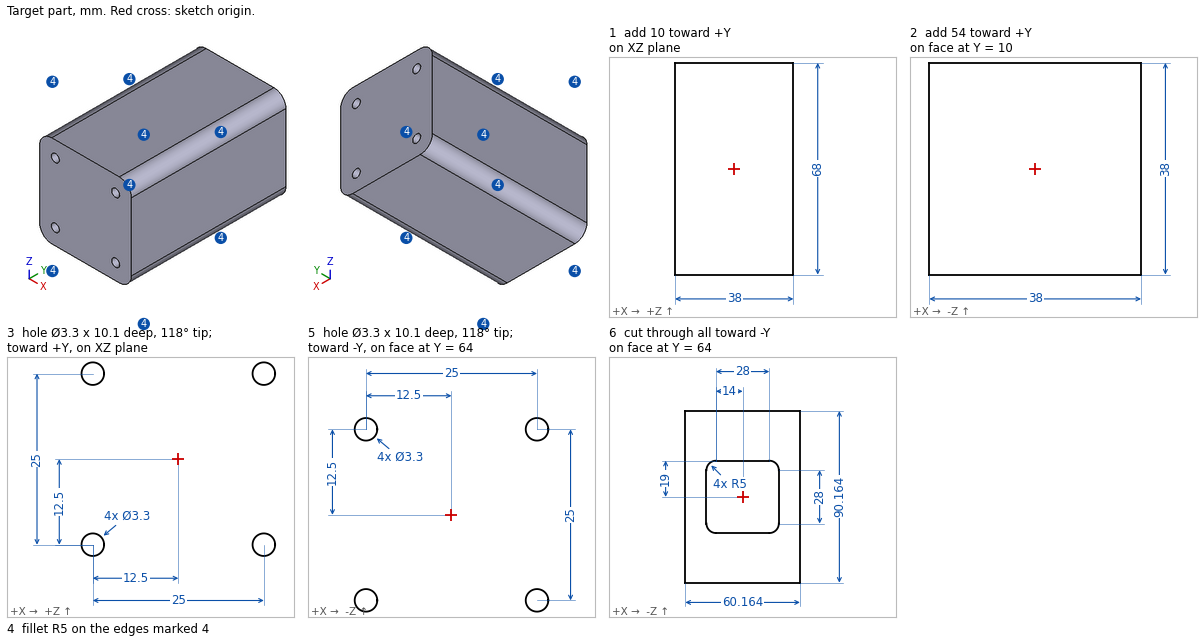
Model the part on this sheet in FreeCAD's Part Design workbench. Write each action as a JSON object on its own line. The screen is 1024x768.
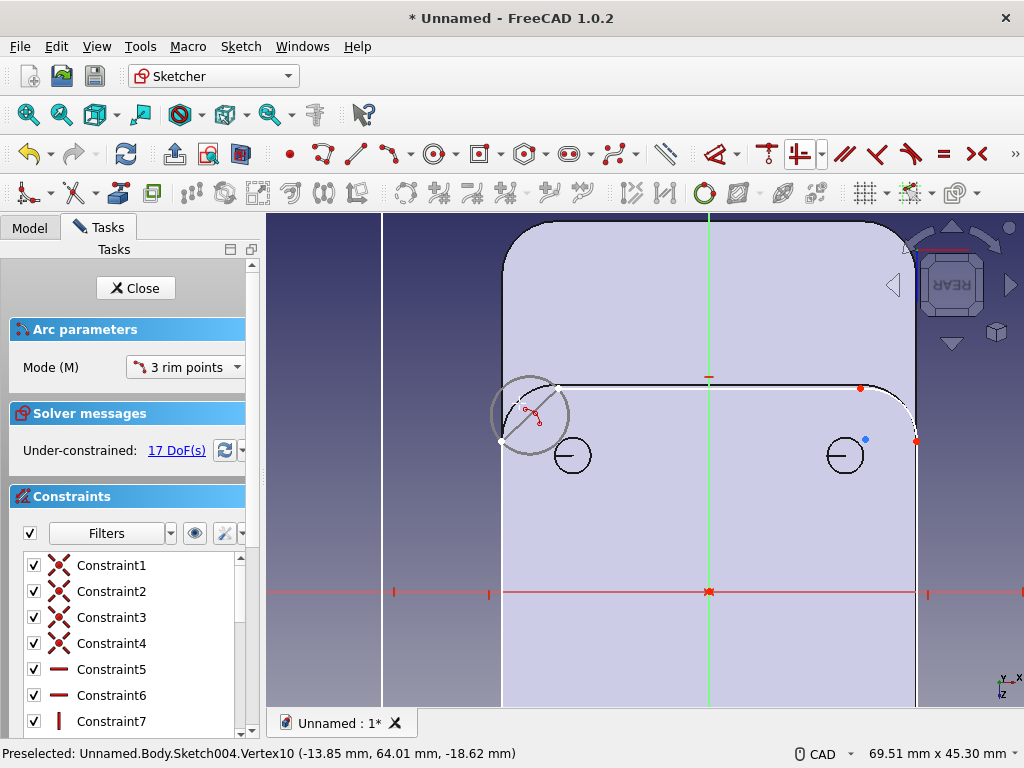
{"action": "left_click", "coordinate": [518, 401]}
{"action": "key", "text": "Escape"}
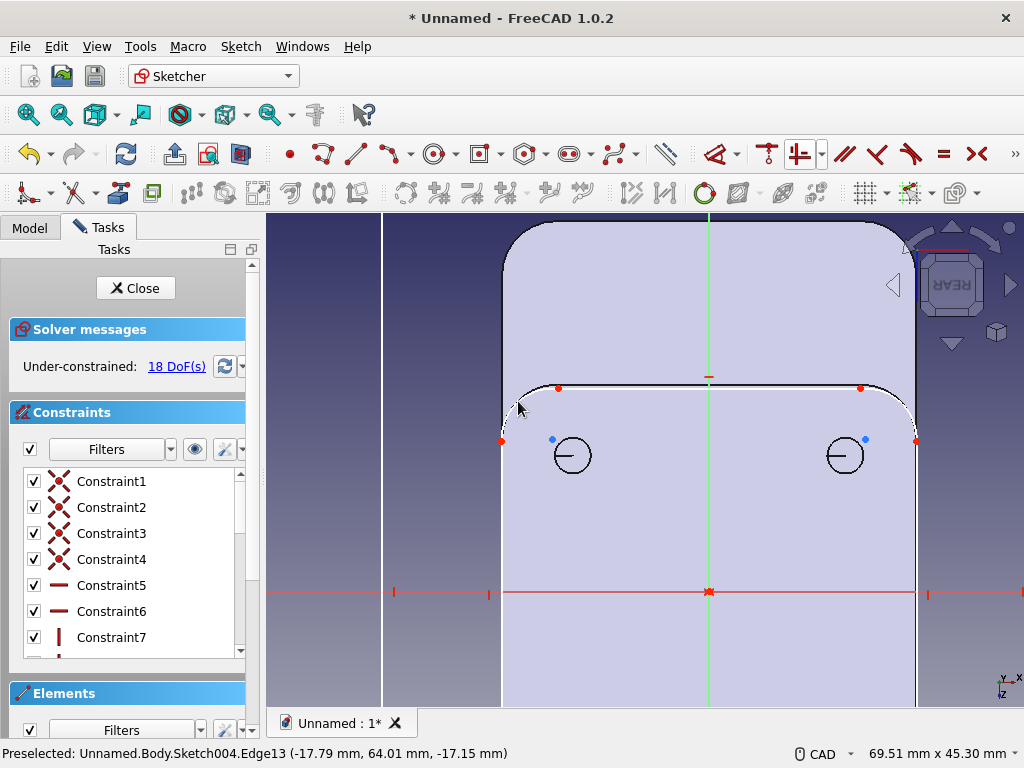
{"action": "left_click", "coordinate": [649, 389]}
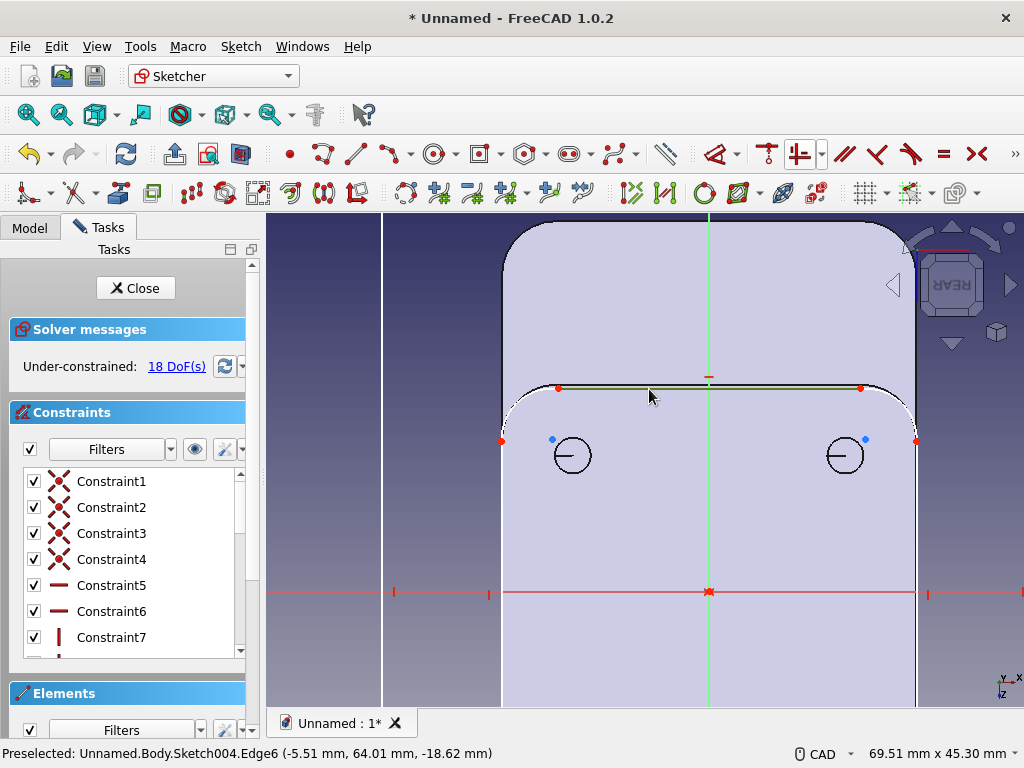
{"action": "scroll", "coordinate": [519, 403], "scroll_direction": "down", "scroll_amount": 6}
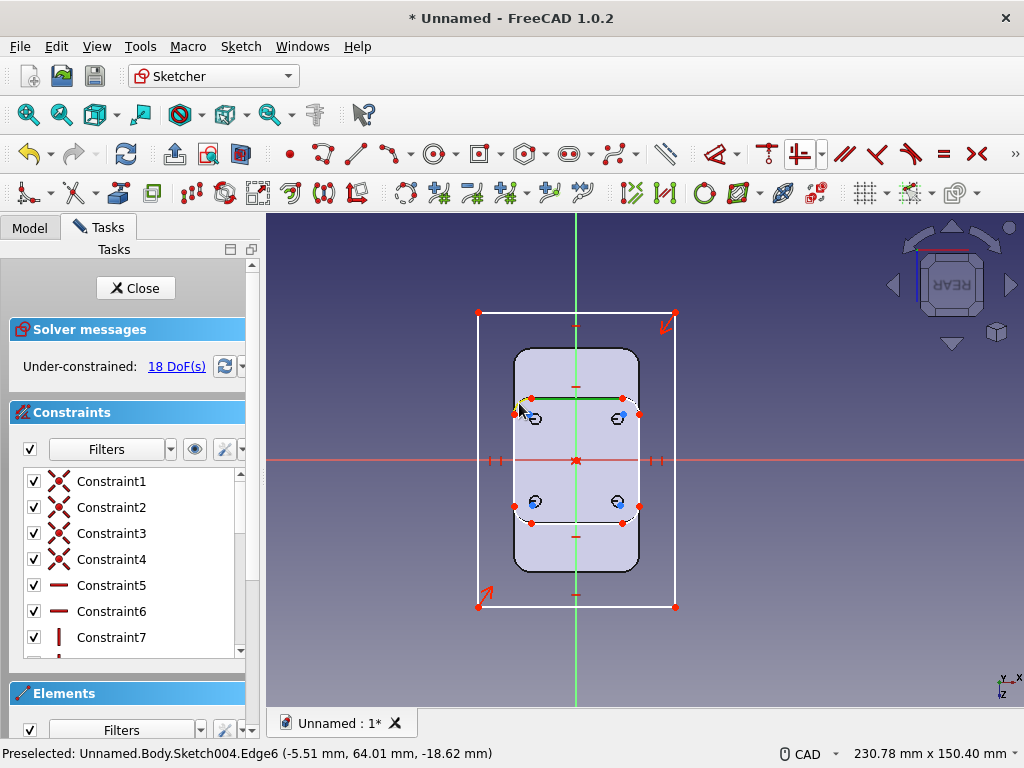
{"action": "scroll", "coordinate": [637, 407], "scroll_direction": "up", "scroll_amount": 3}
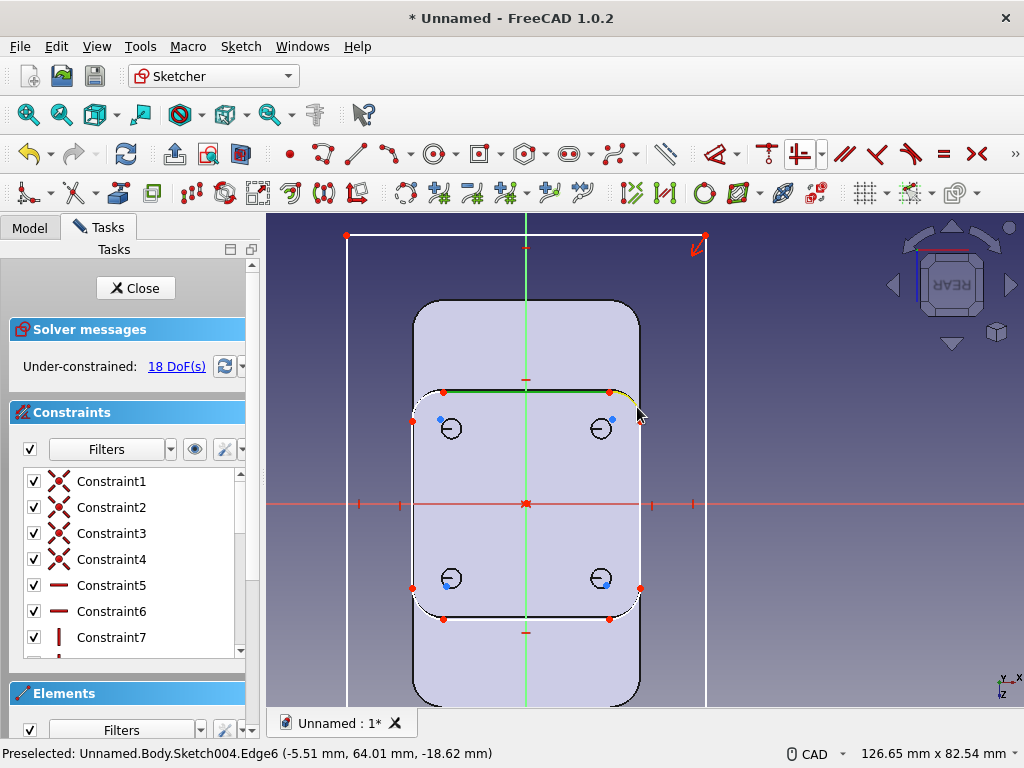
{"action": "left_click", "coordinate": [637, 407]}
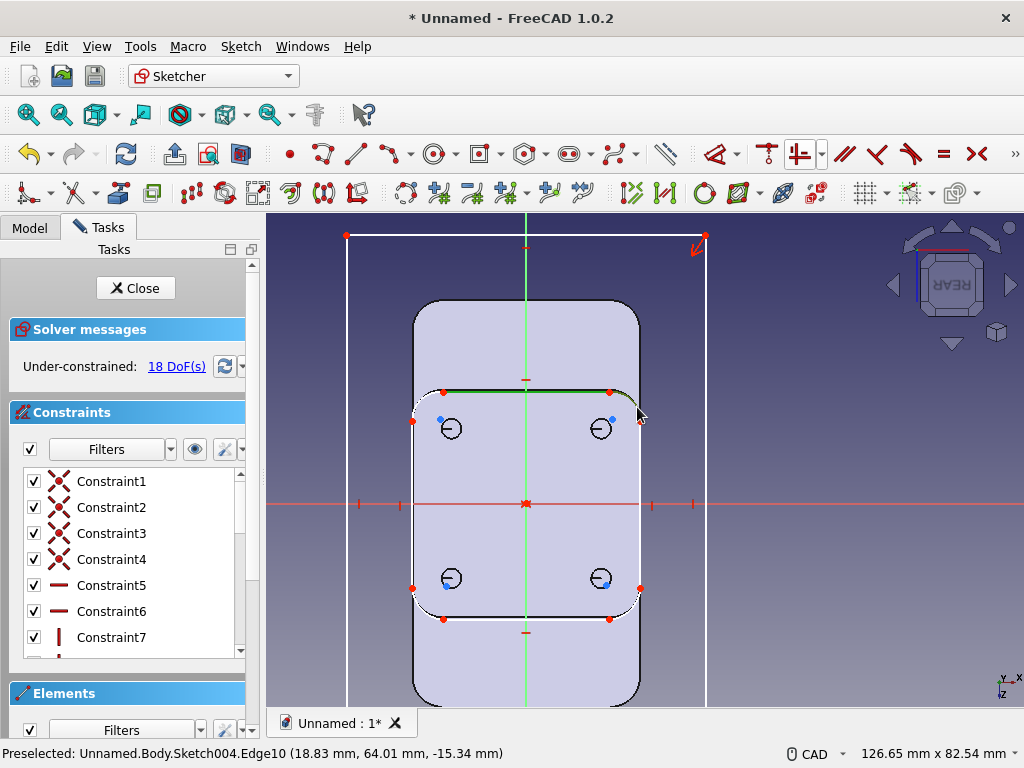
{"action": "left_click", "coordinate": [911, 154]}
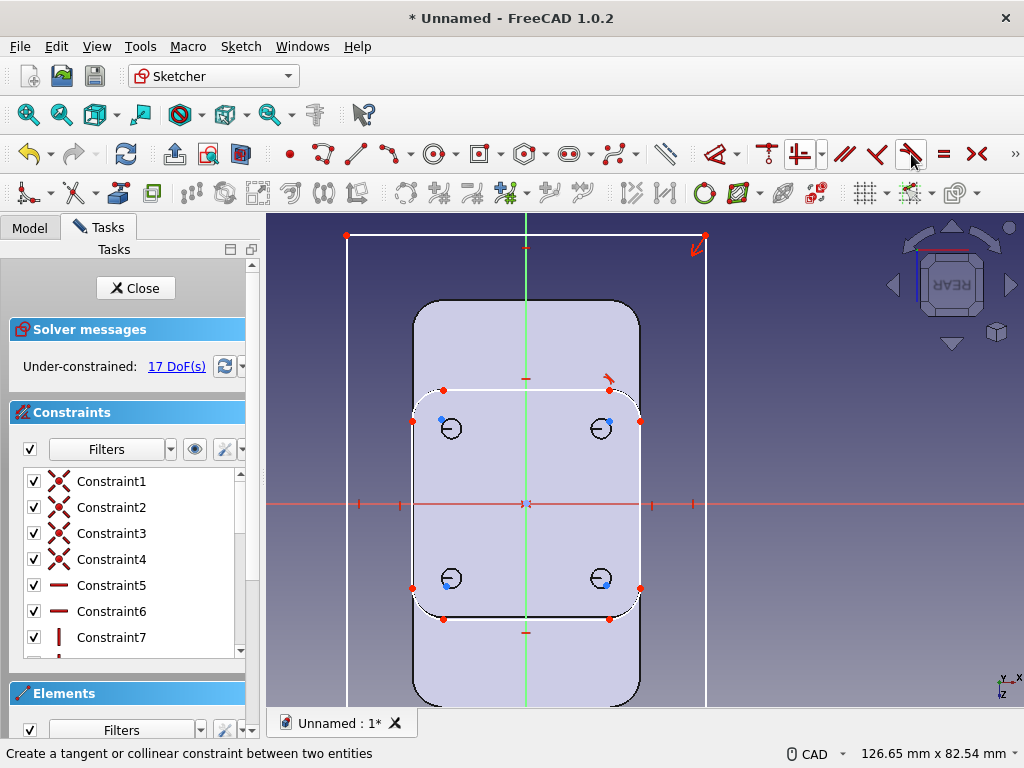
{"action": "left_click", "coordinate": [493, 390]}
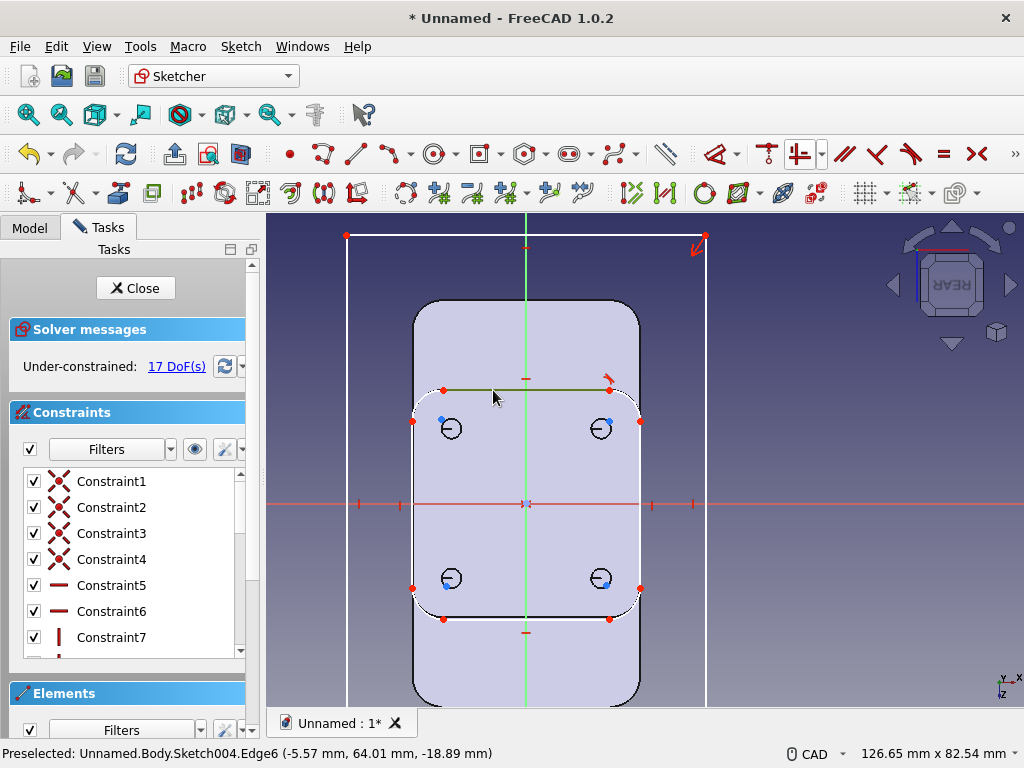
{"action": "left_click", "coordinate": [429, 393]}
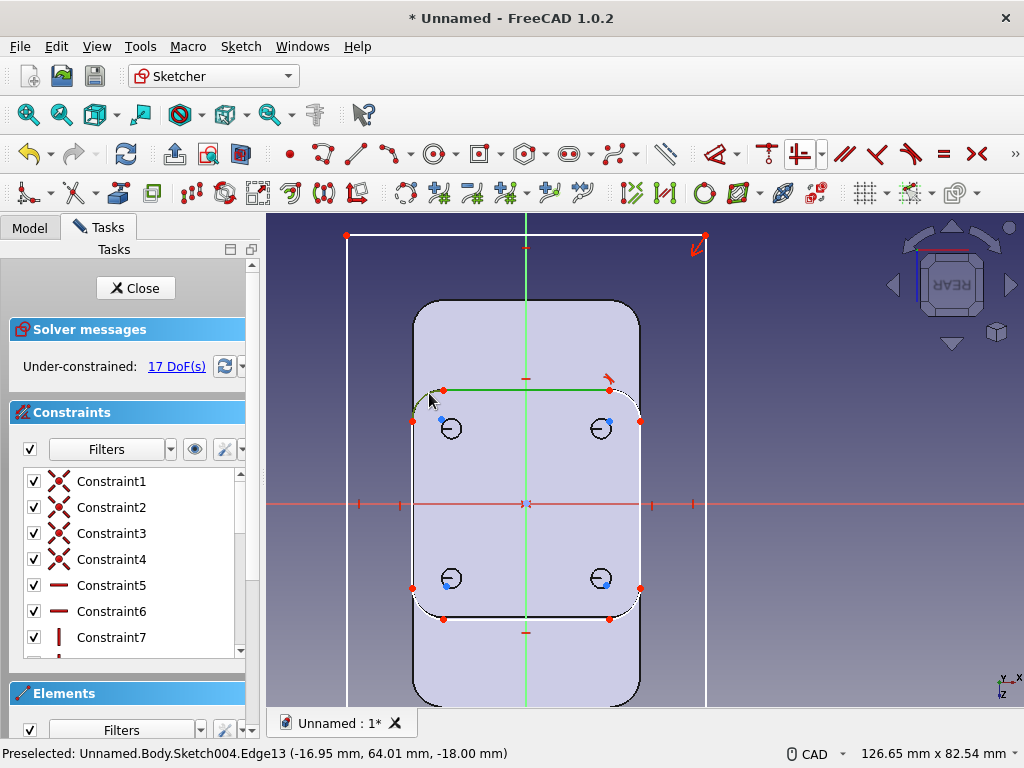
{"action": "left_click", "coordinate": [911, 154]}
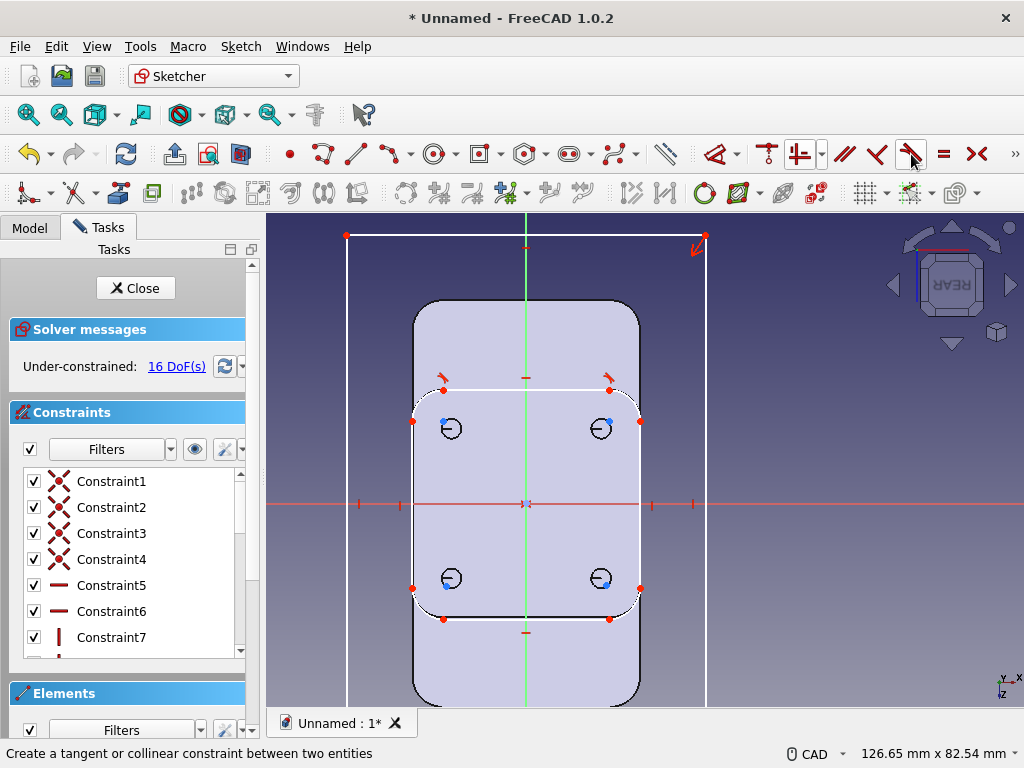
{"action": "left_click", "coordinate": [640, 472]}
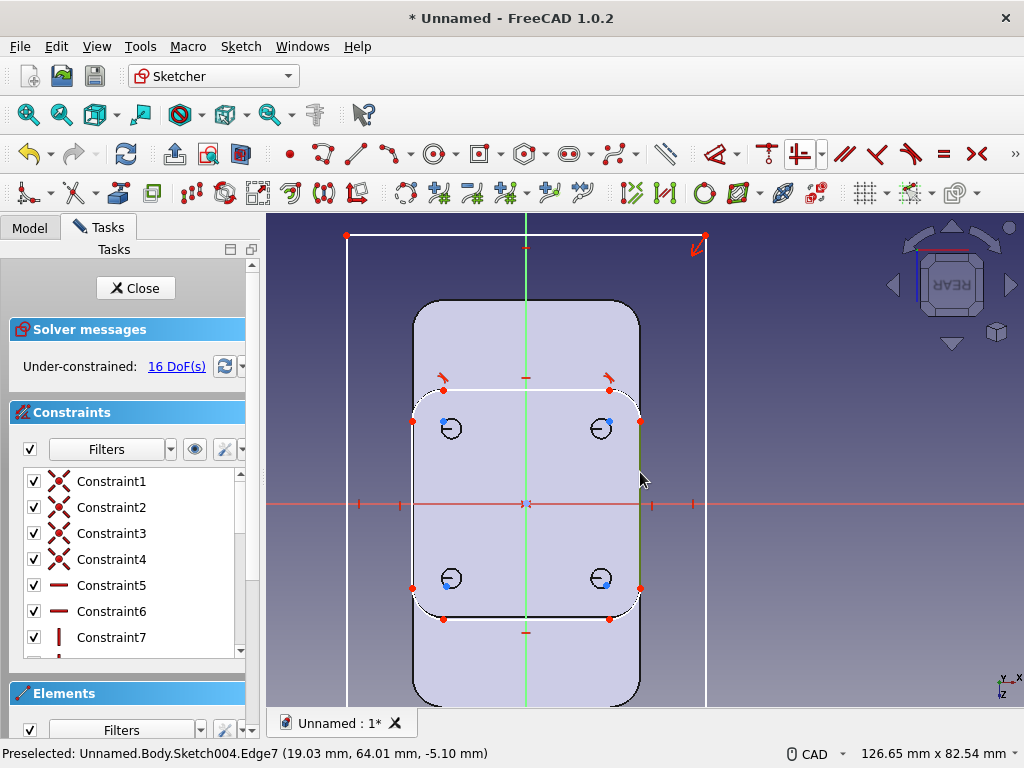
{"action": "left_click", "coordinate": [637, 407]}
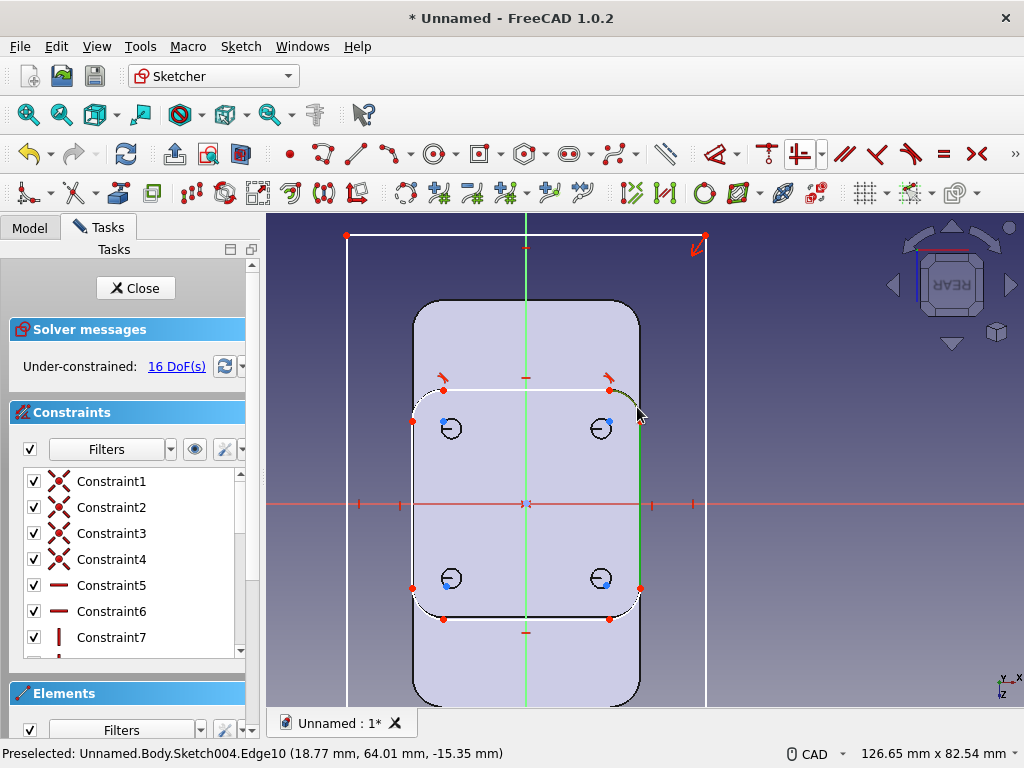
{"action": "left_click", "coordinate": [911, 154]}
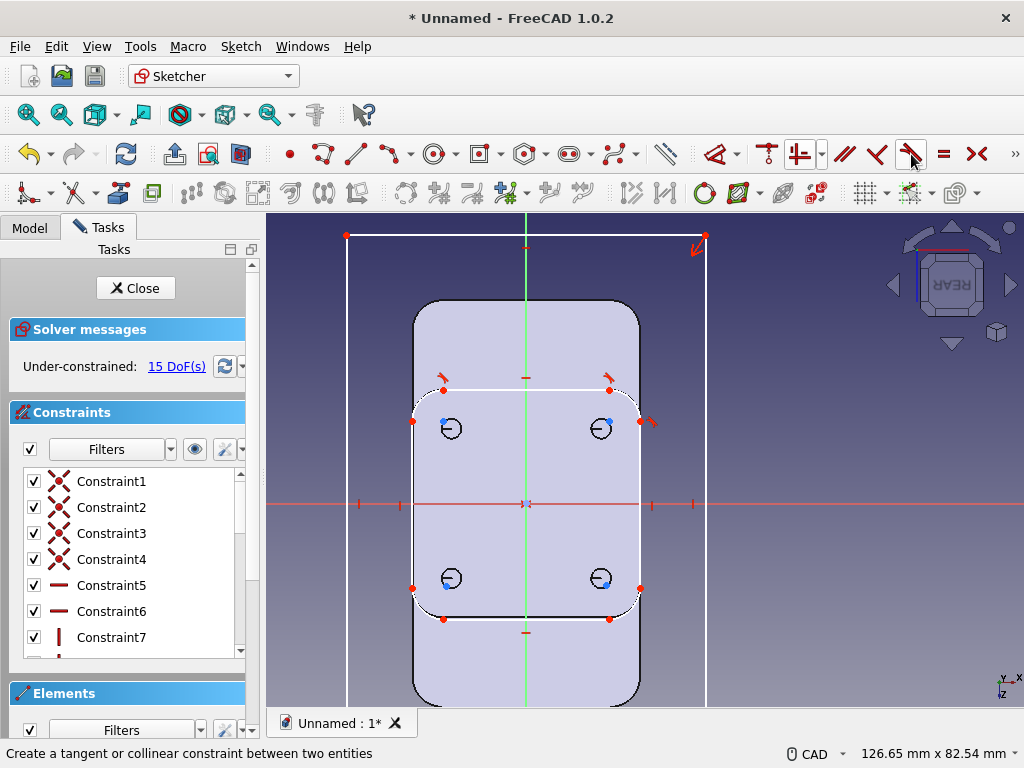
{"action": "left_click", "coordinate": [640, 472]}